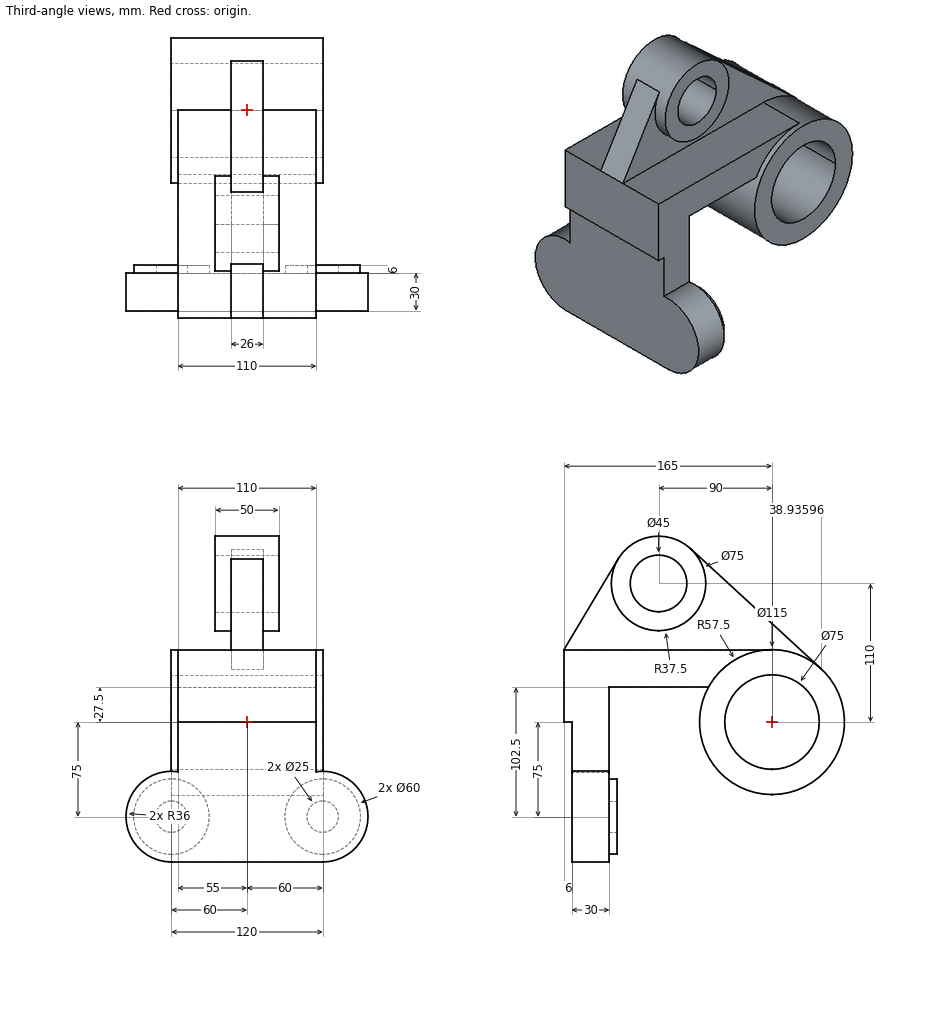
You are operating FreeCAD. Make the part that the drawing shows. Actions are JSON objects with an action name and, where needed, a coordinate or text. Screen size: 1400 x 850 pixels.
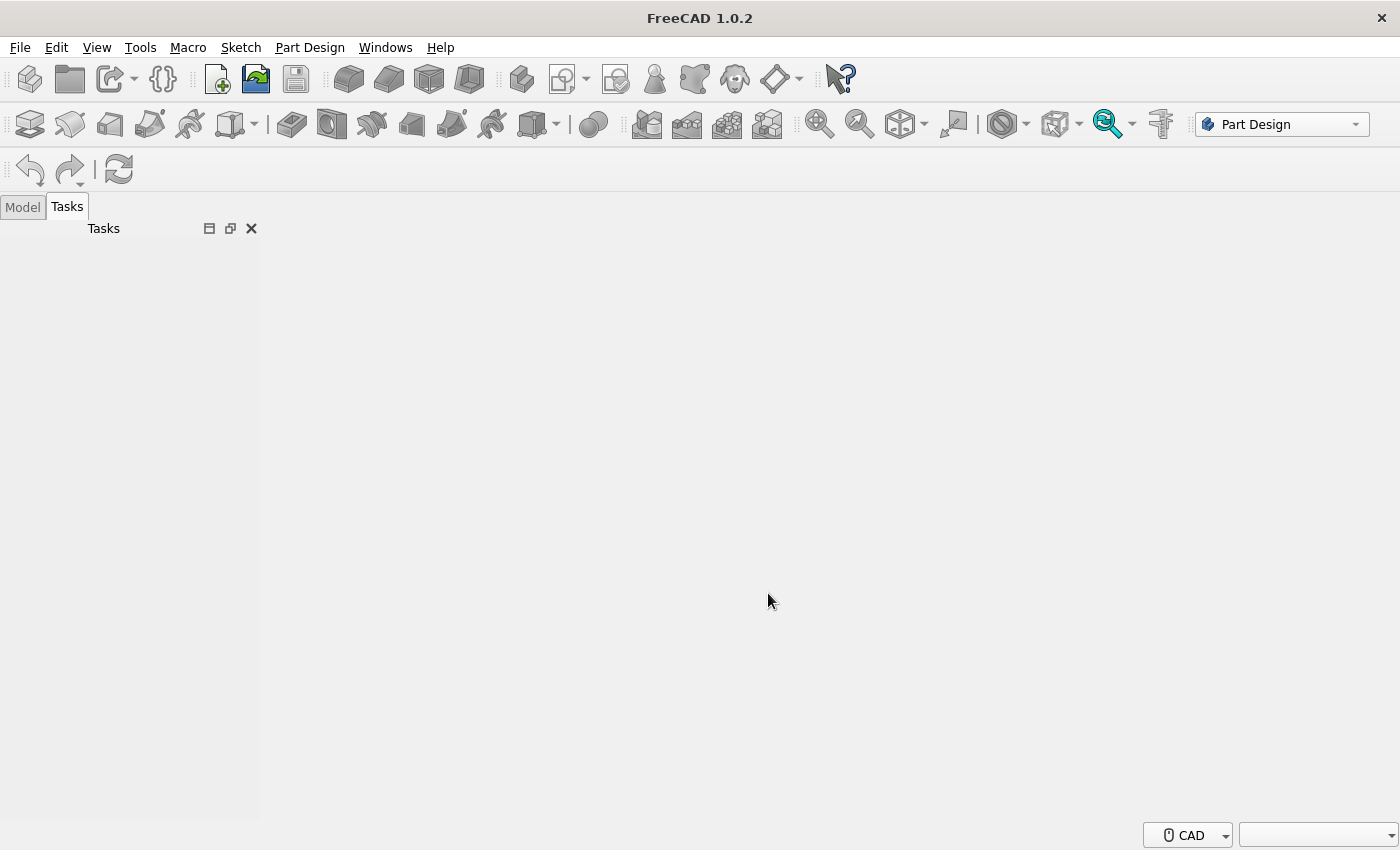
{"action": "left_click", "coordinate": [216, 80]}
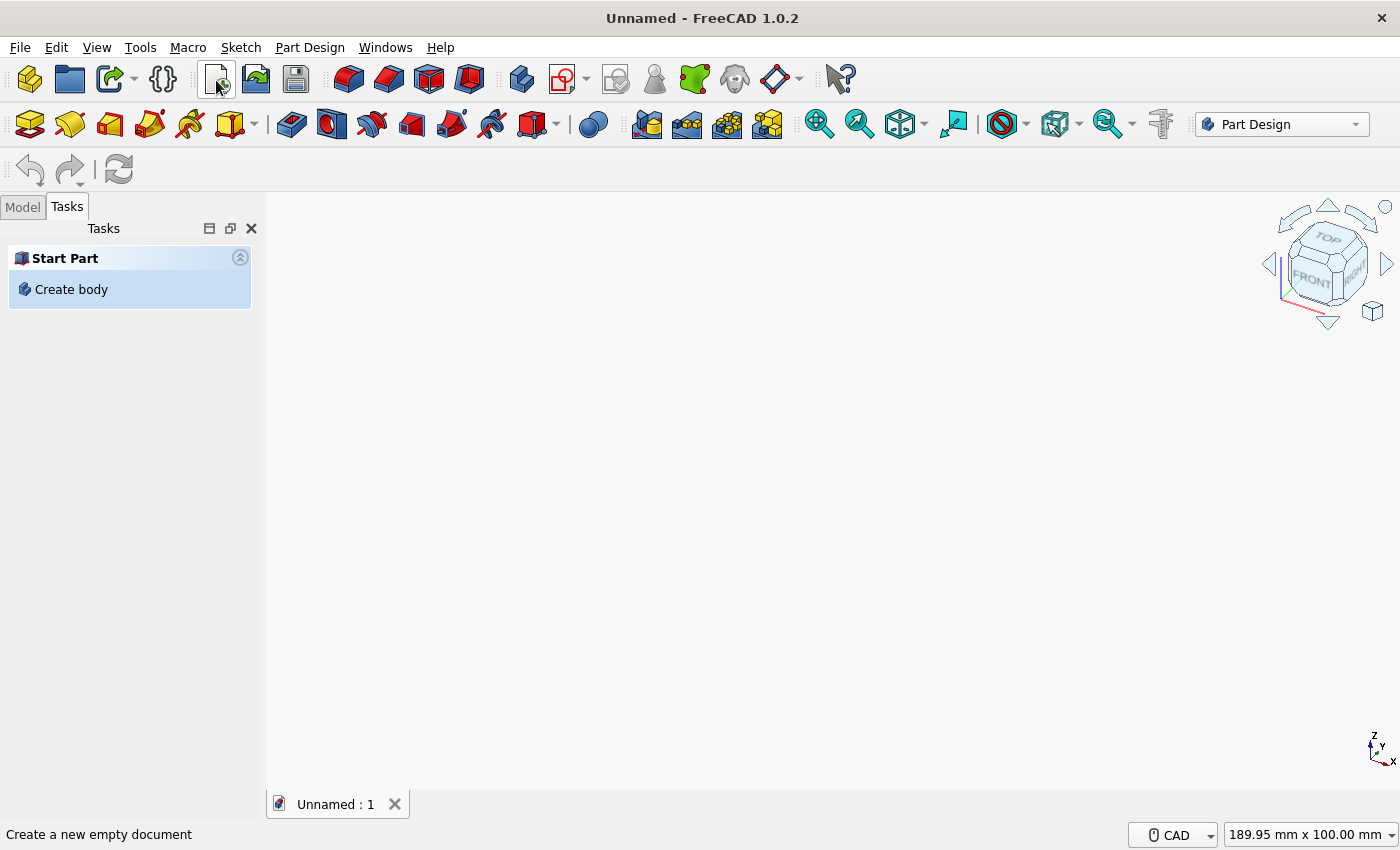
{"action": "left_click", "coordinate": [562, 80]}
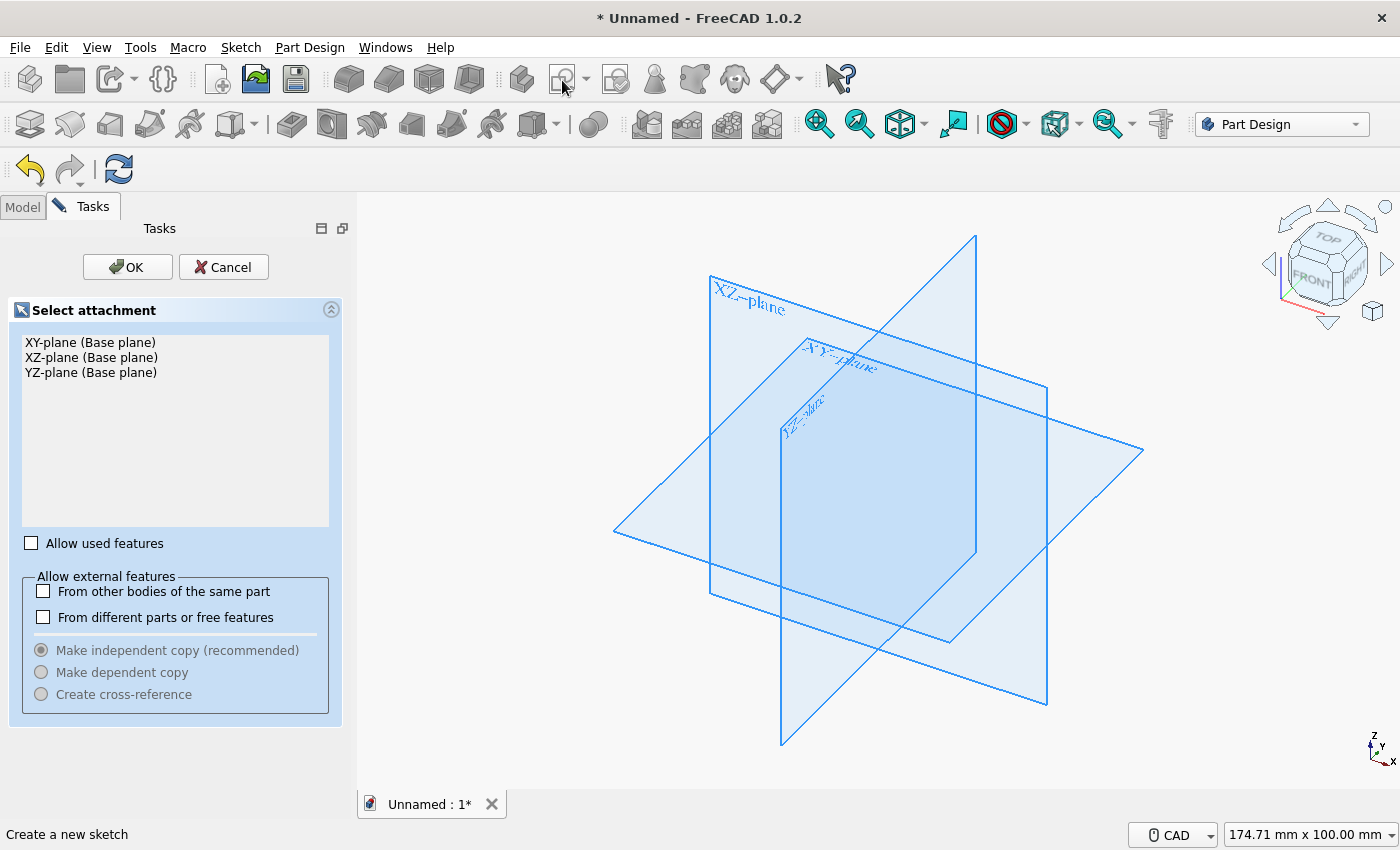
{"action": "left_click", "coordinate": [82, 372]}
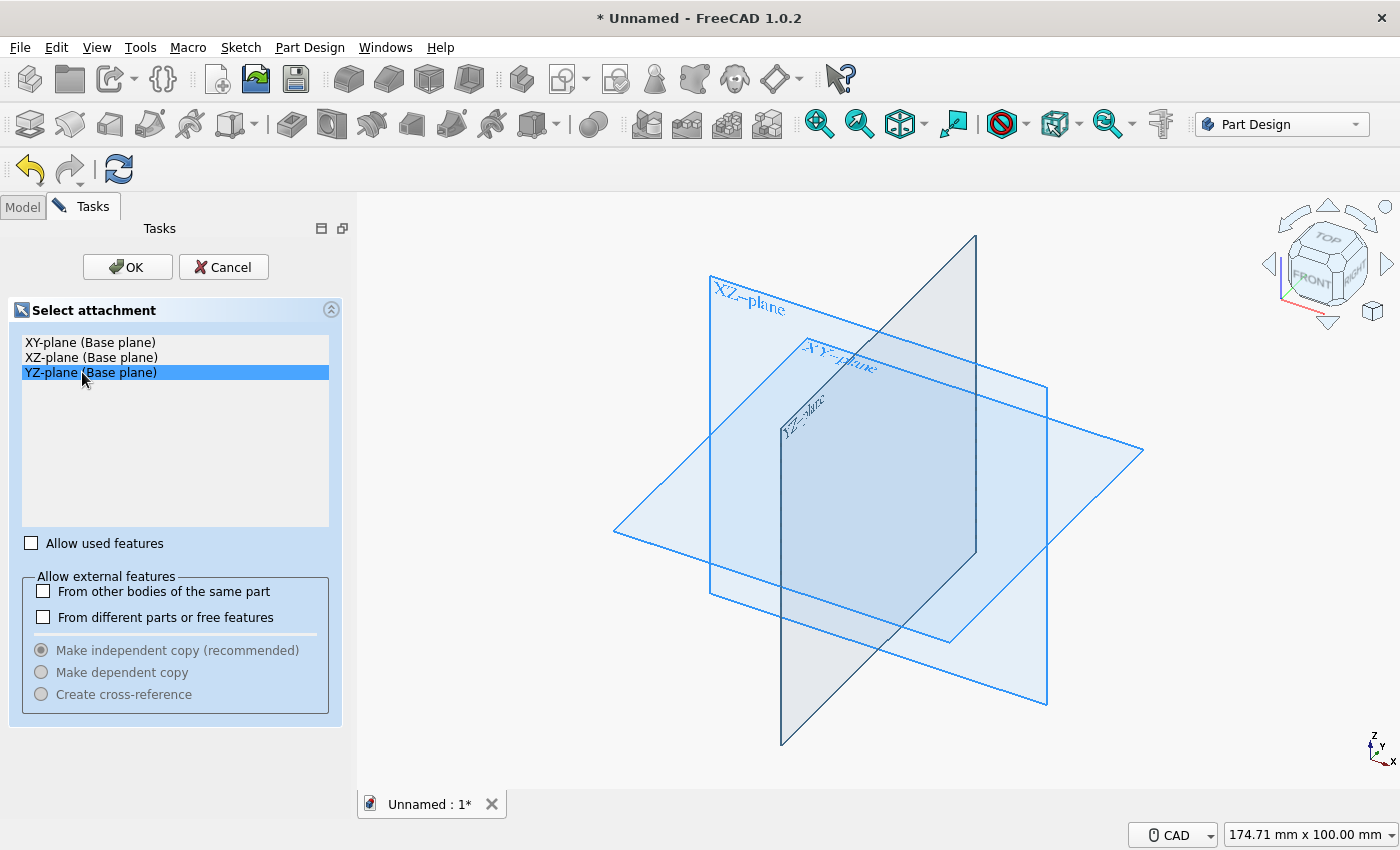
{"action": "left_click", "coordinate": [128, 267]}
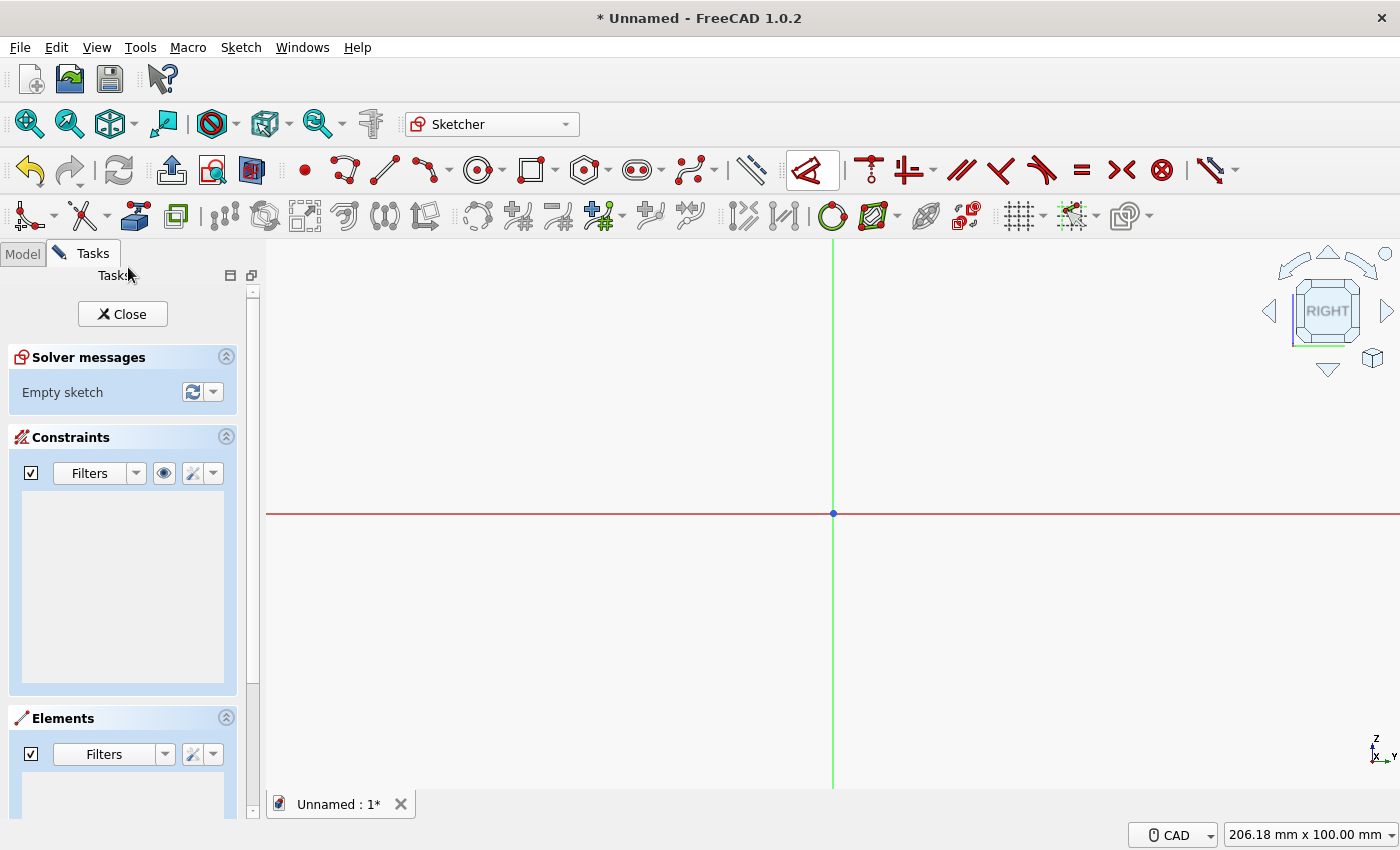
{"action": "scroll", "coordinate": [681, 514], "scroll_direction": "down", "scroll_amount": 3}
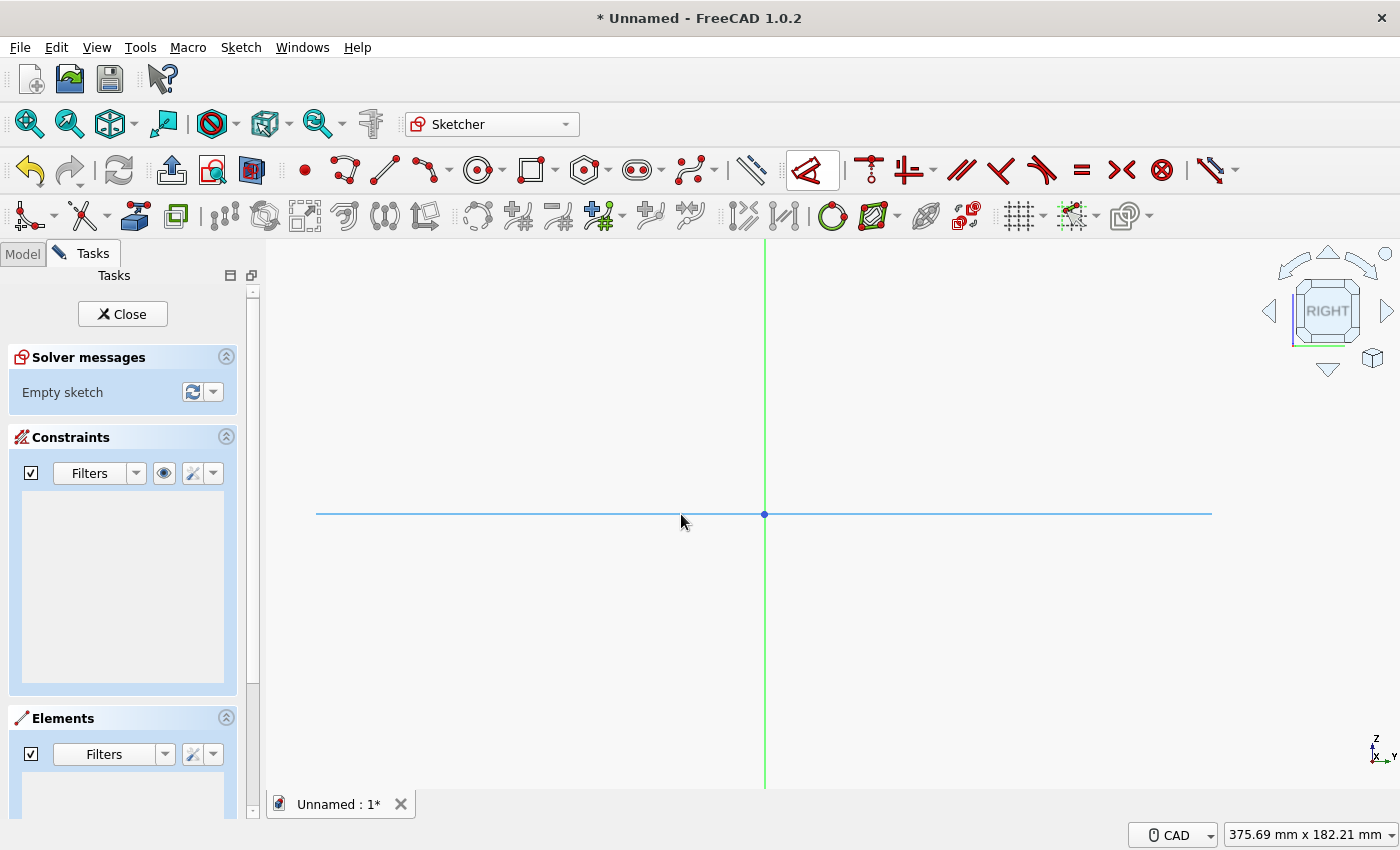
{"action": "left_click", "coordinate": [478, 170]}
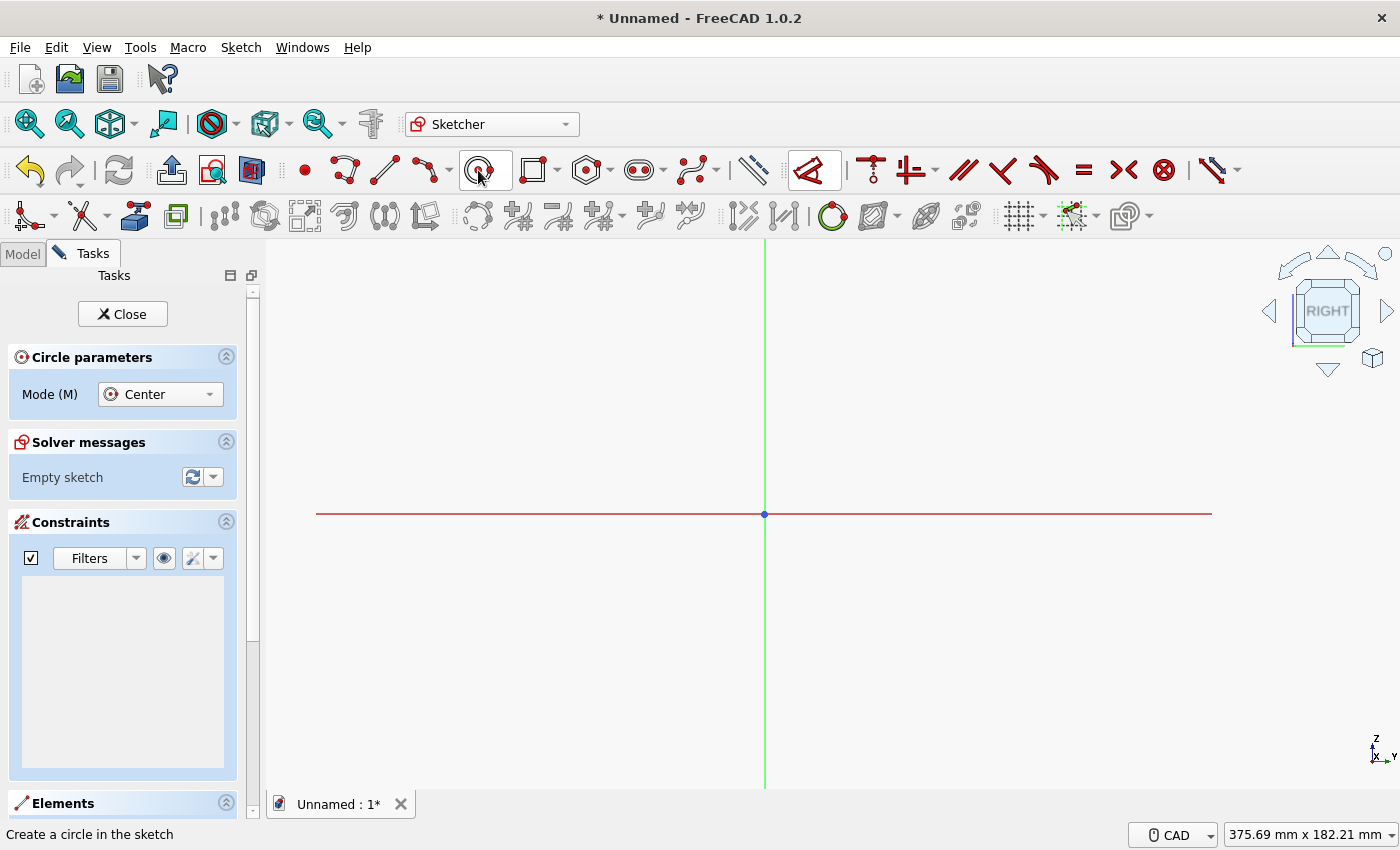
{"action": "left_click", "coordinate": [765, 514]}
{"action": "mouse_move", "coordinate": [887, 391]}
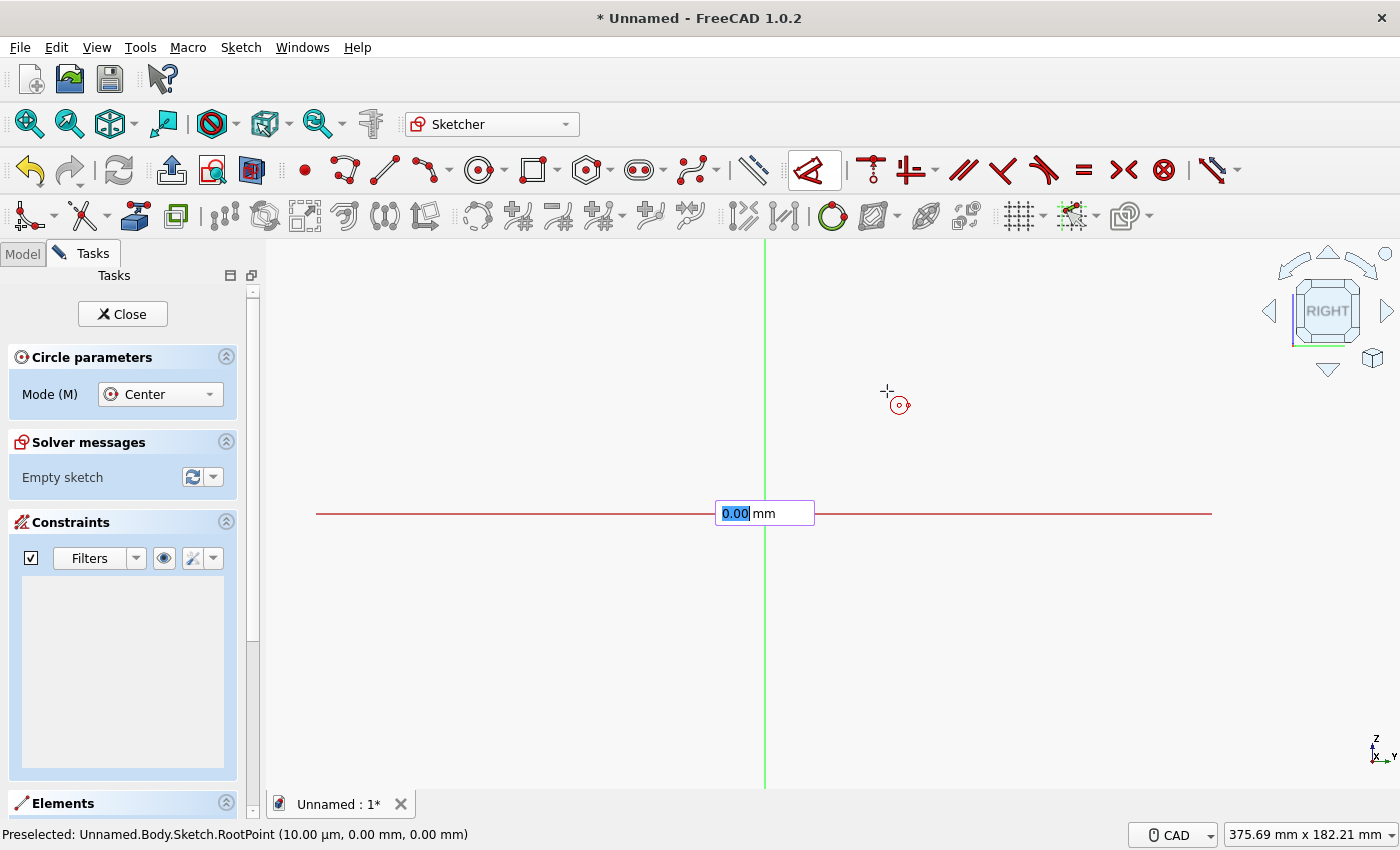
{"action": "type", "text": "115"}
{"action": "key", "text": "Return"}